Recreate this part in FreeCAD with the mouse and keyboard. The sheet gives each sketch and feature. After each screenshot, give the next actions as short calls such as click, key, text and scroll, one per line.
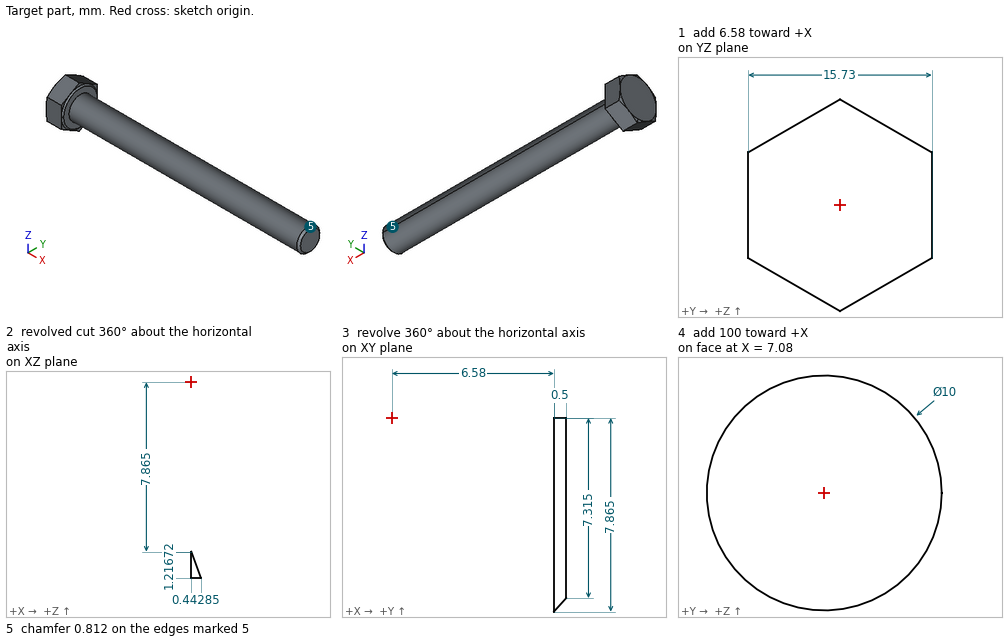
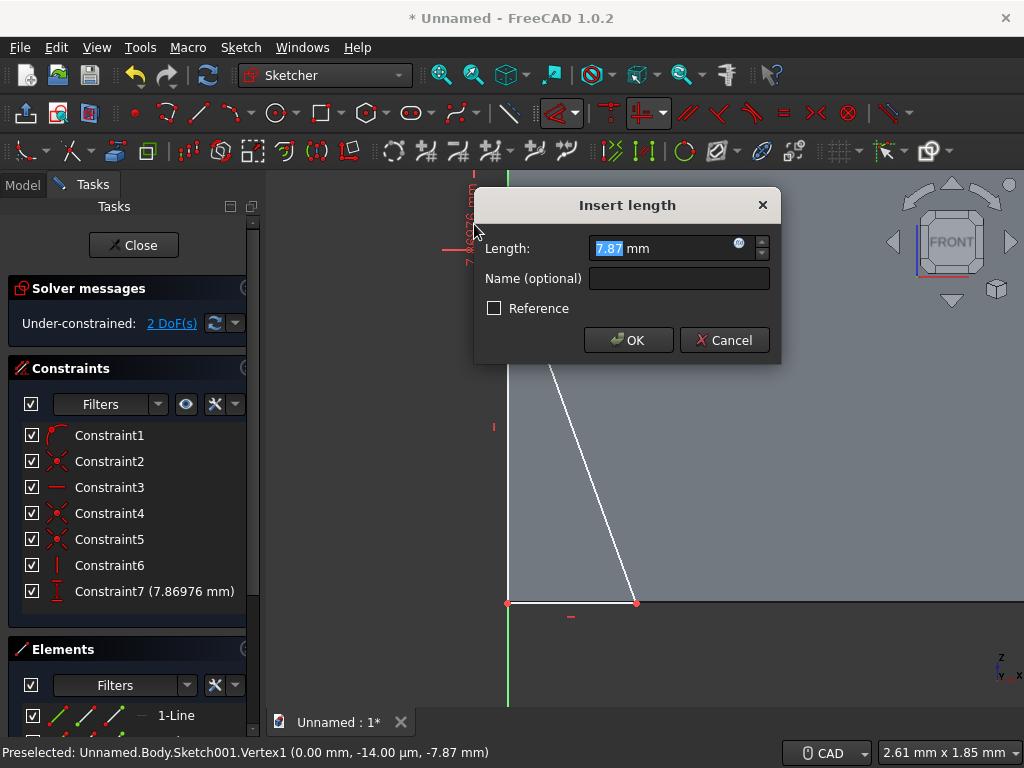
text(7.865)
key(Return)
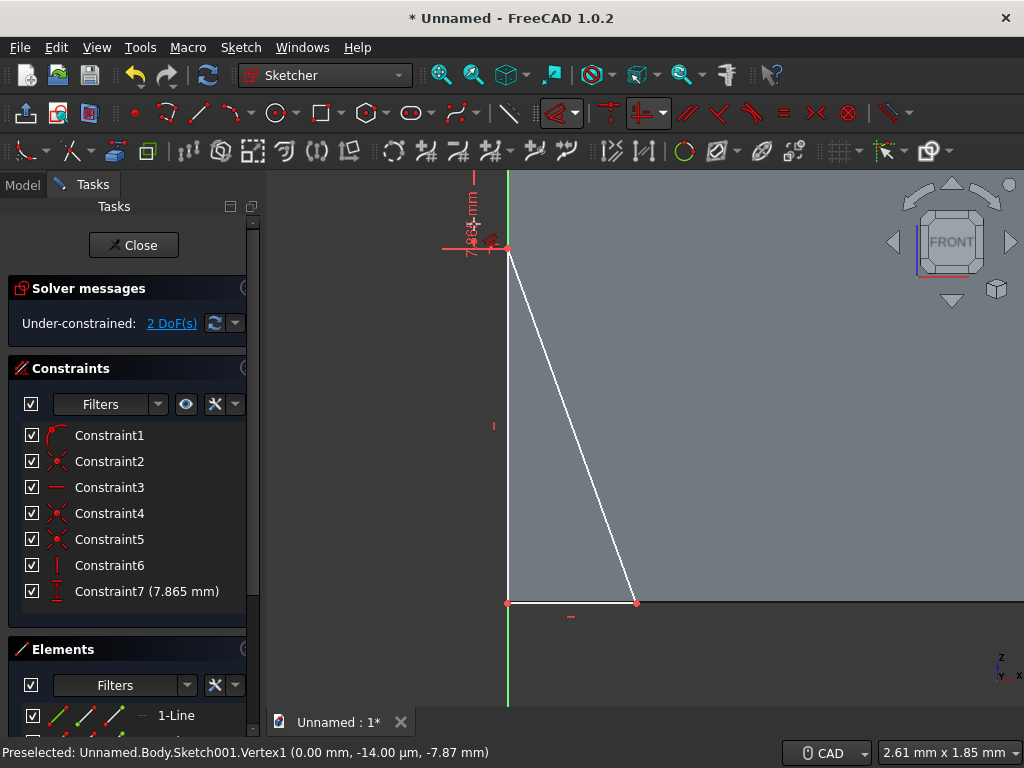
click(597, 603)
click(572, 637)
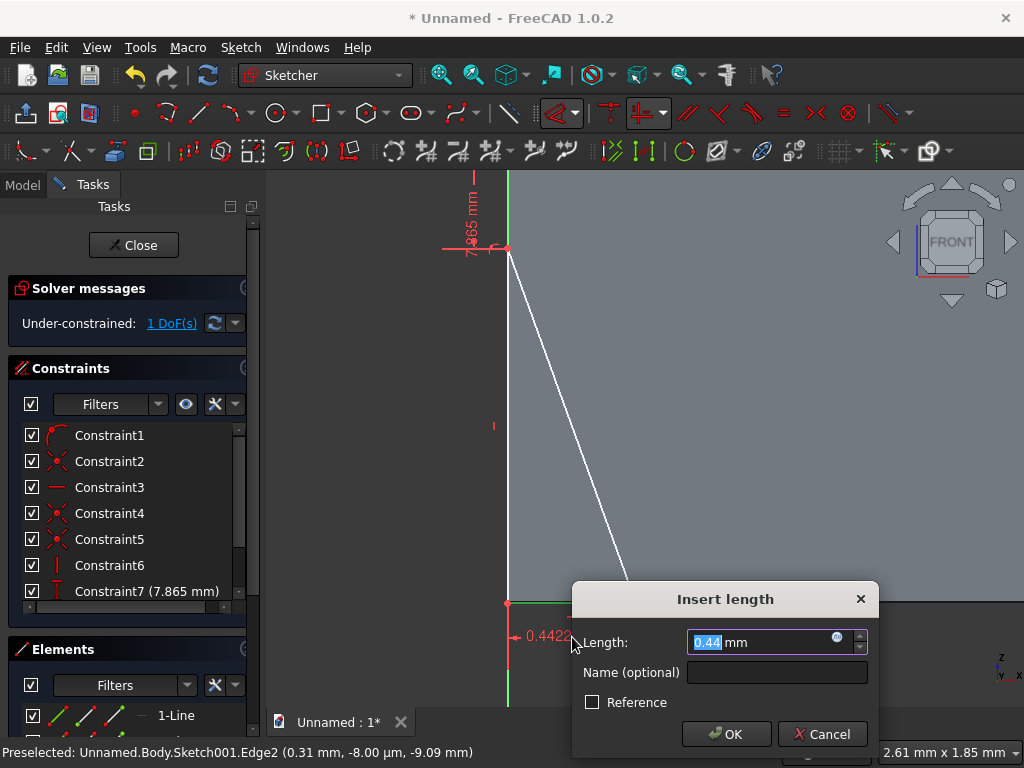
text(0.44285)
key(Return)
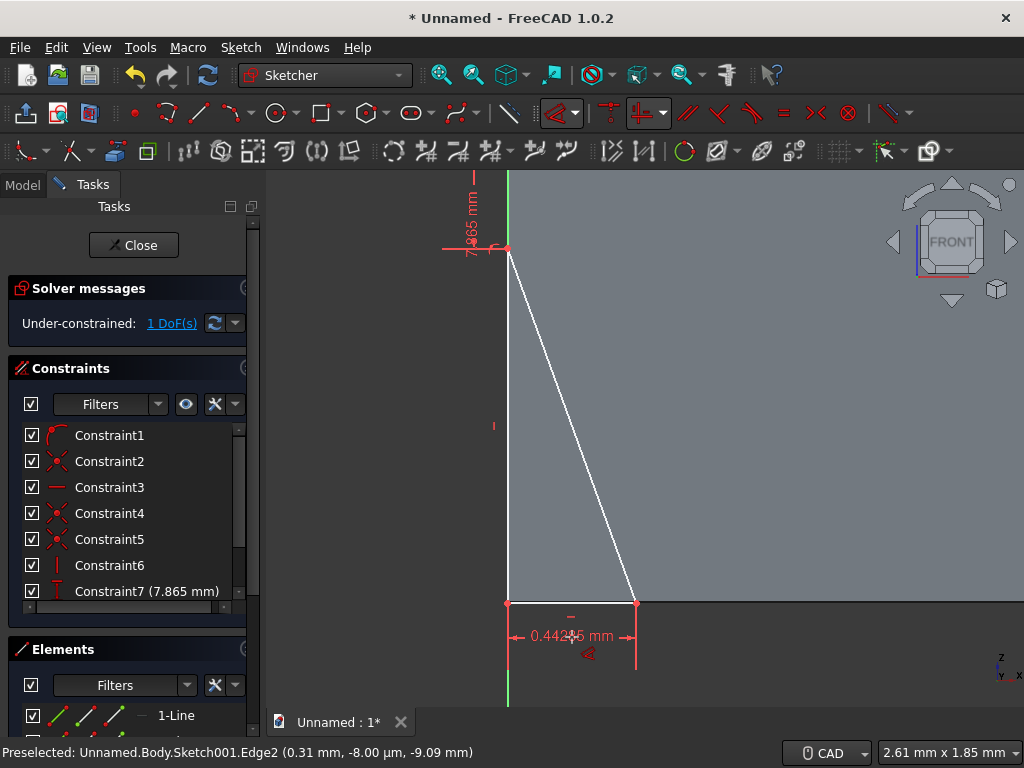
click(508, 497)
click(474, 426)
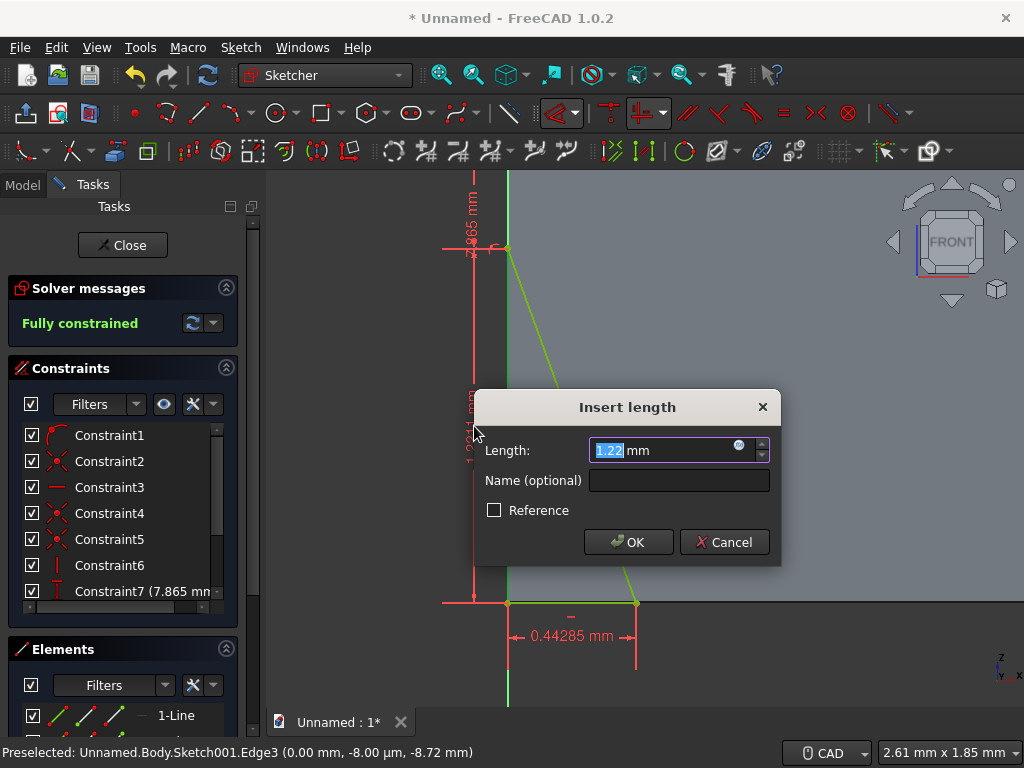
text(1.21672)
key(Return)
key(Escape)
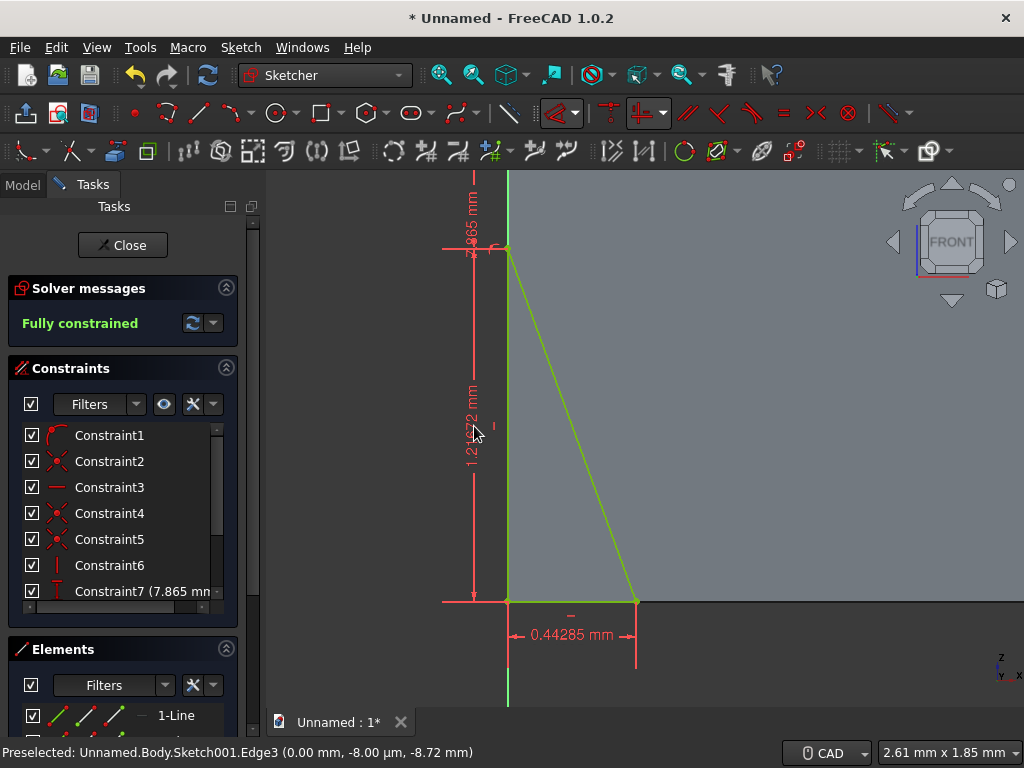
click(123, 245)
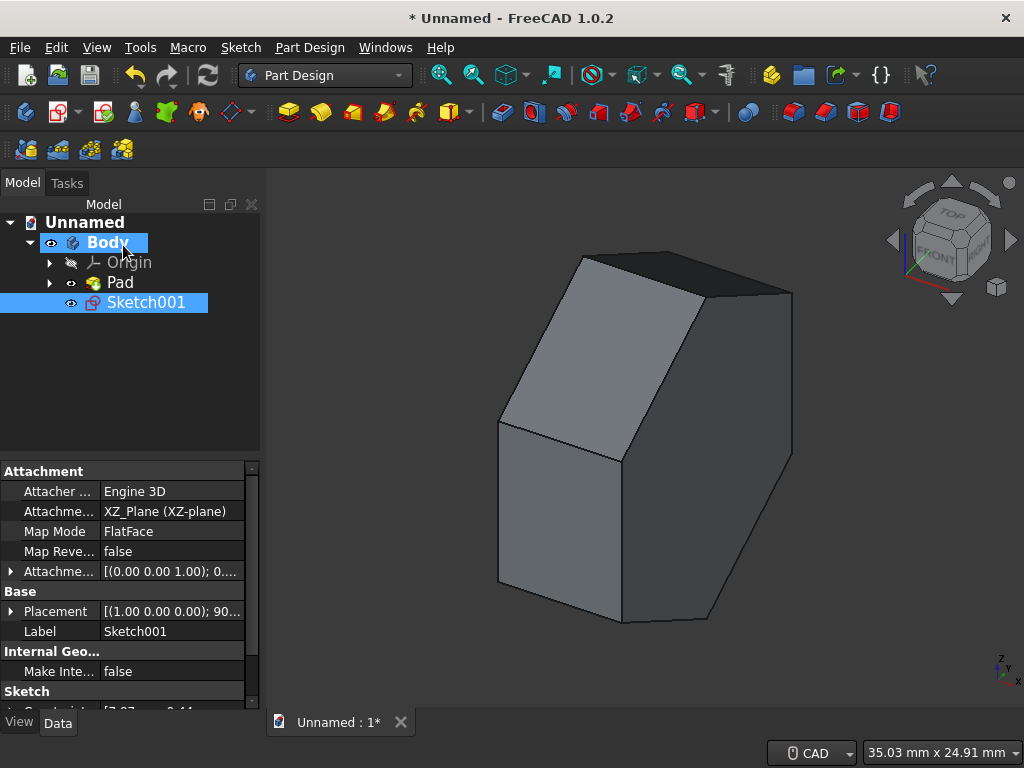
click(568, 112)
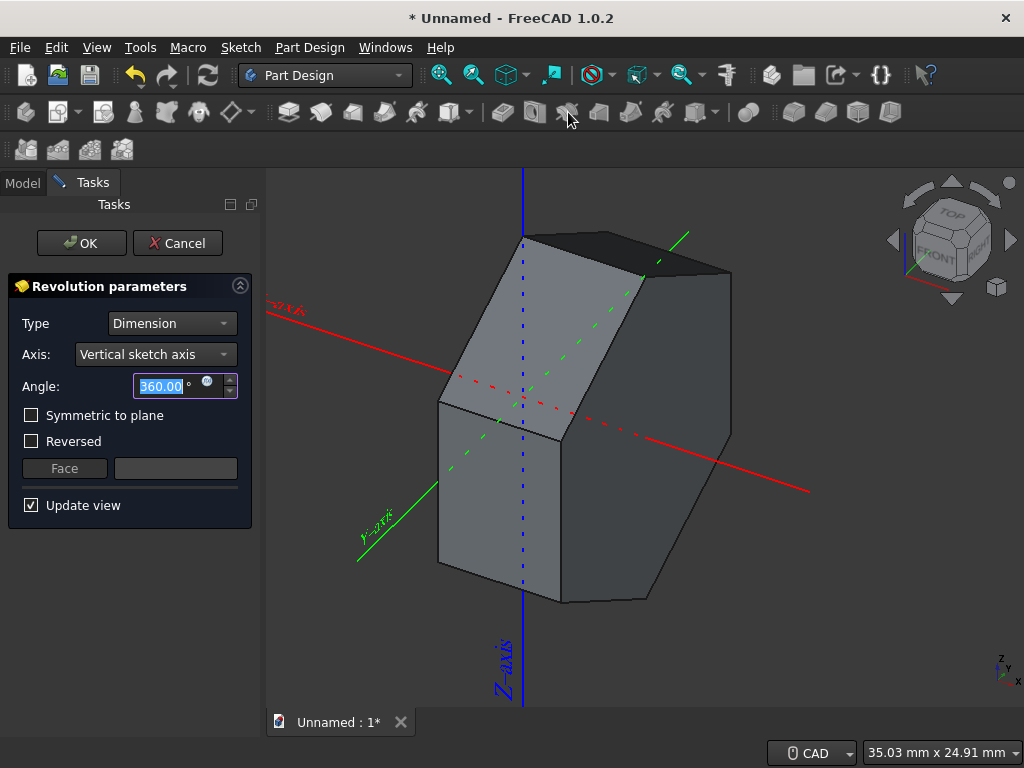
click(156, 354)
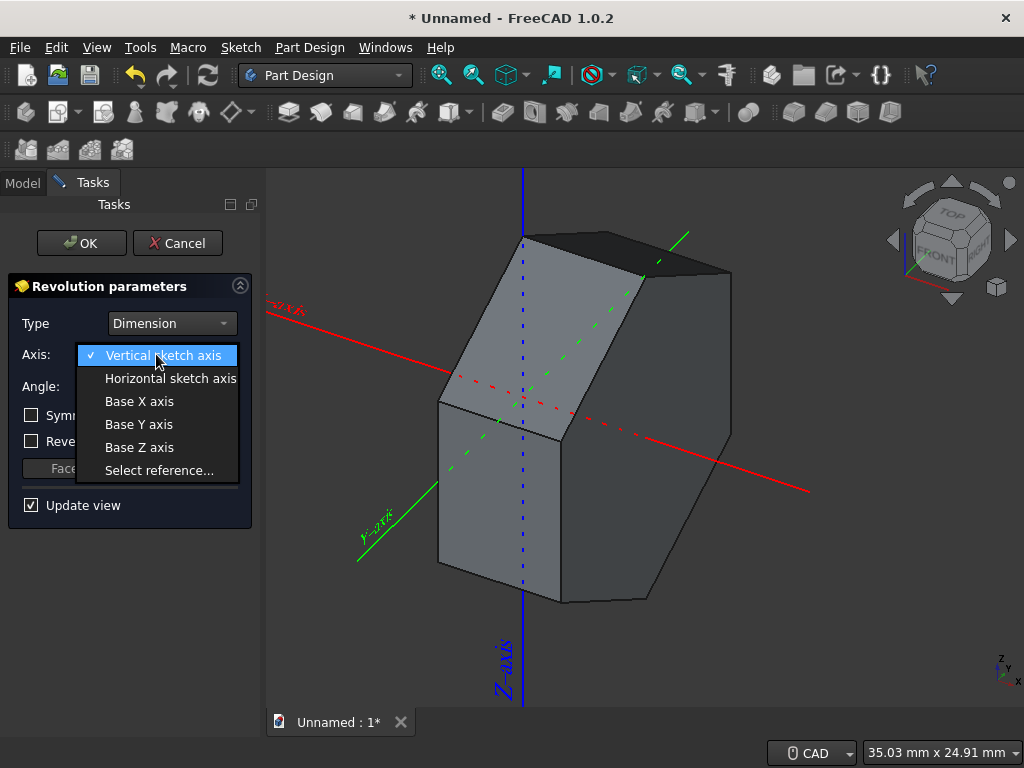
click(156, 378)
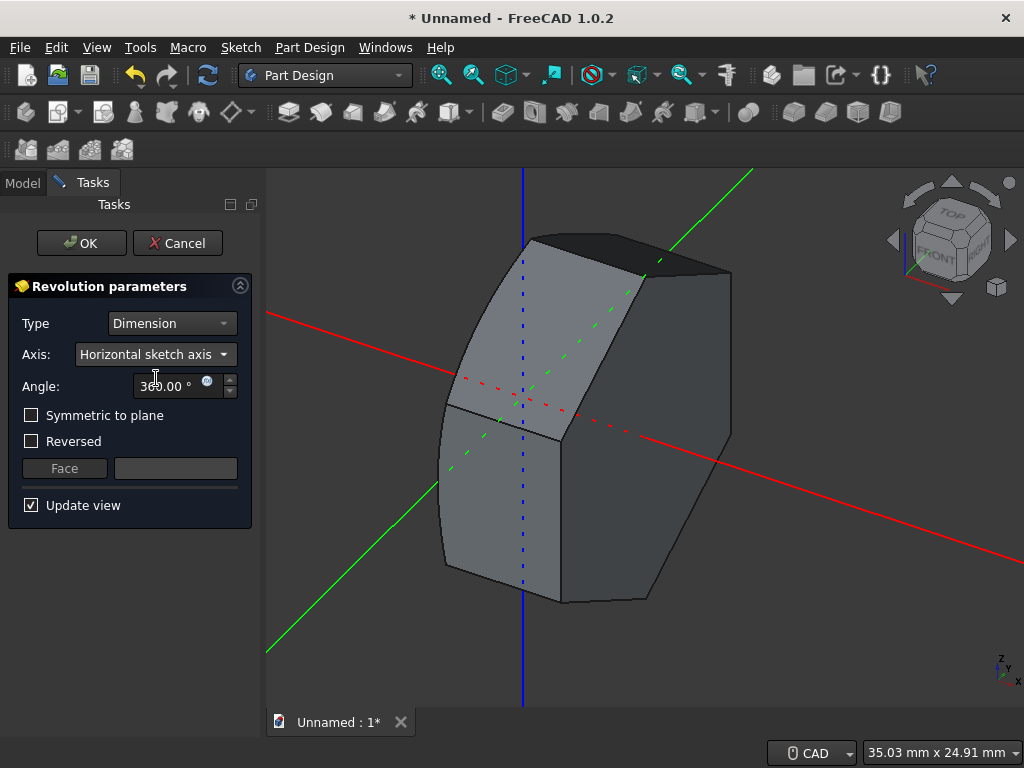
click(82, 243)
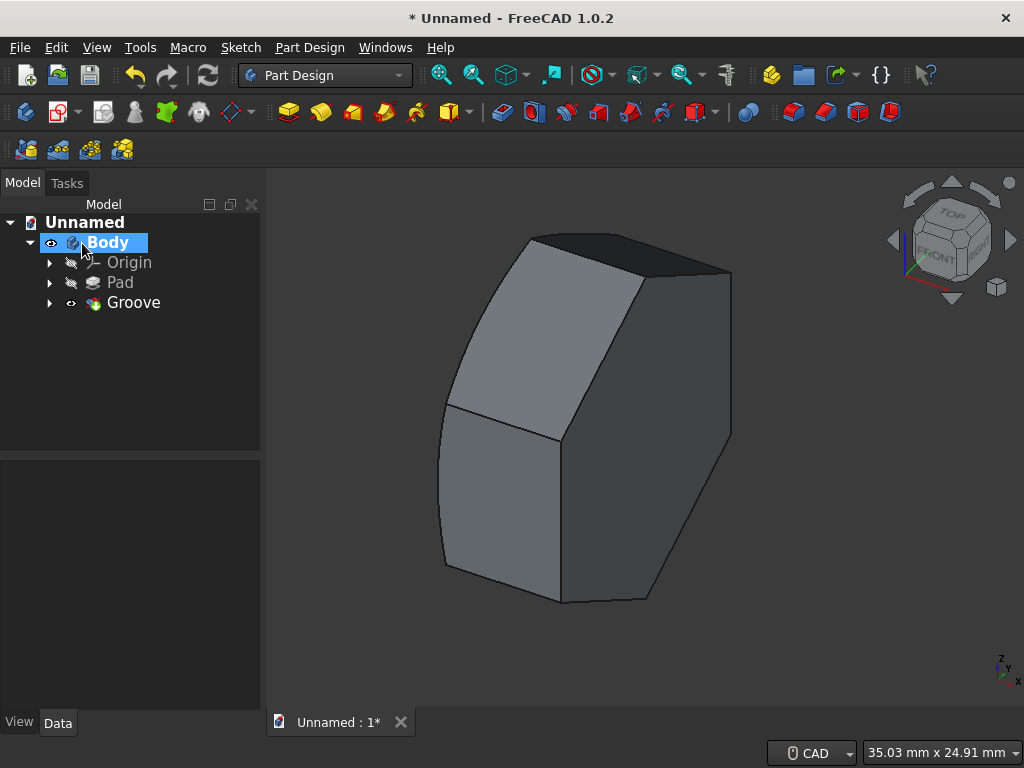
click(442, 76)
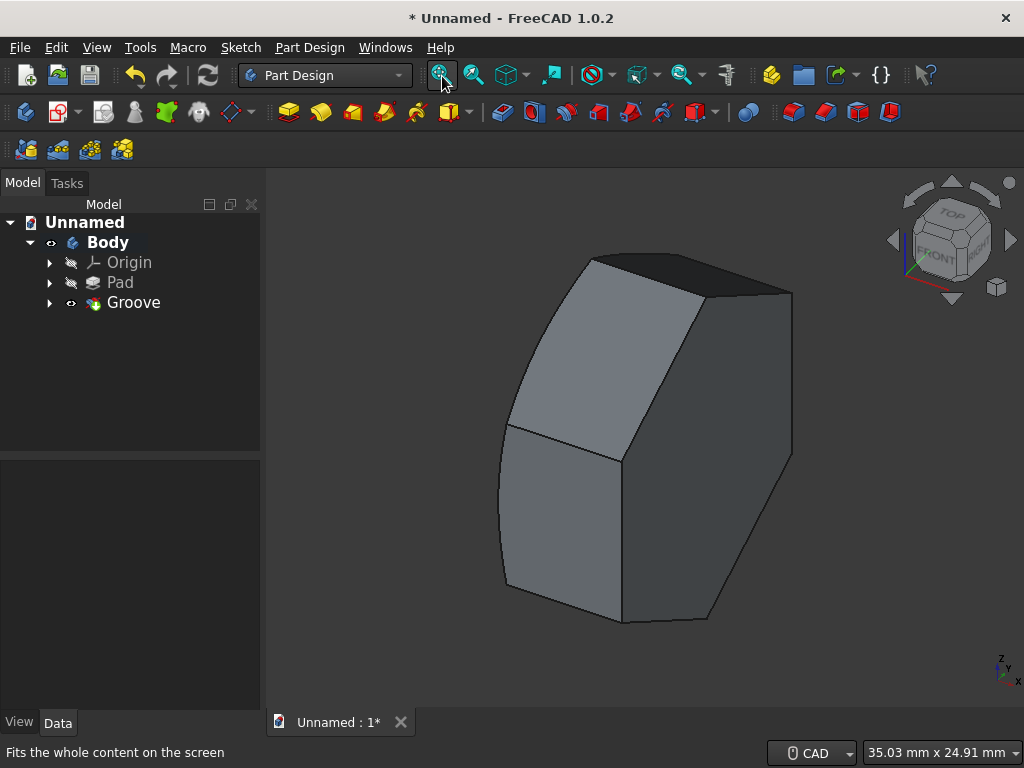
click(58, 112)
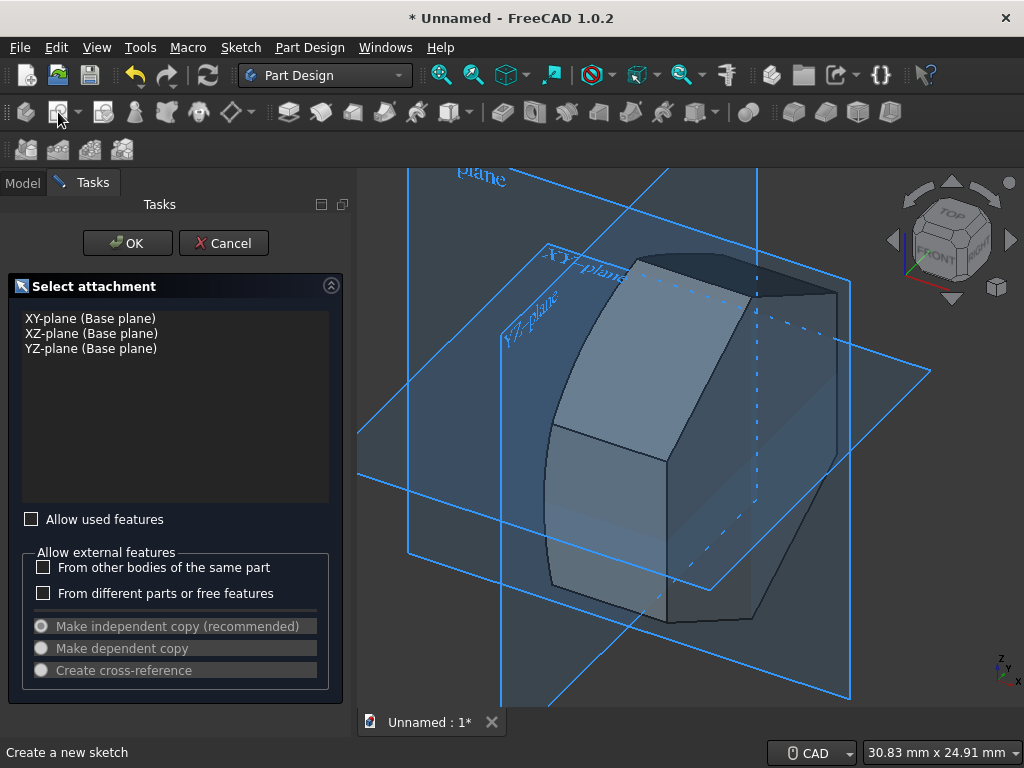
click(82, 318)